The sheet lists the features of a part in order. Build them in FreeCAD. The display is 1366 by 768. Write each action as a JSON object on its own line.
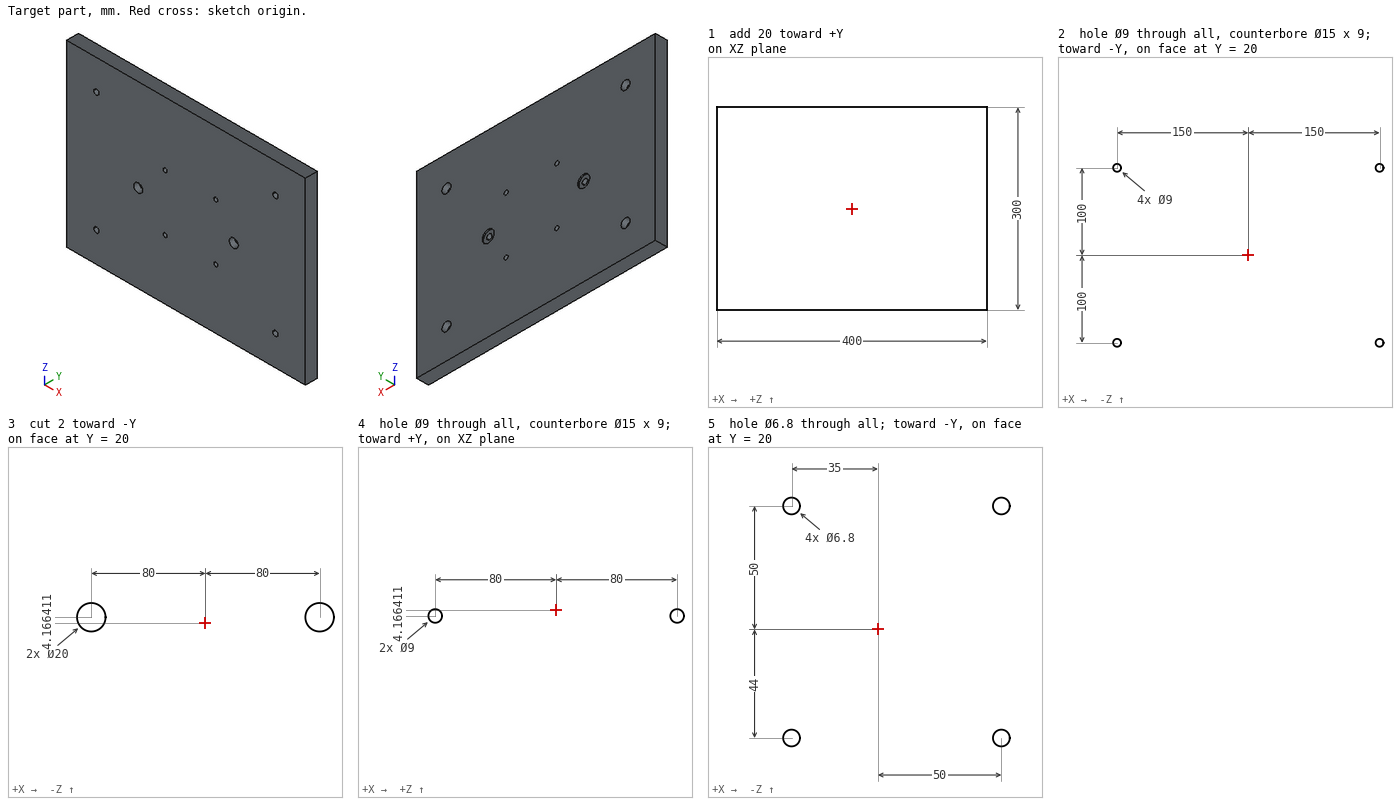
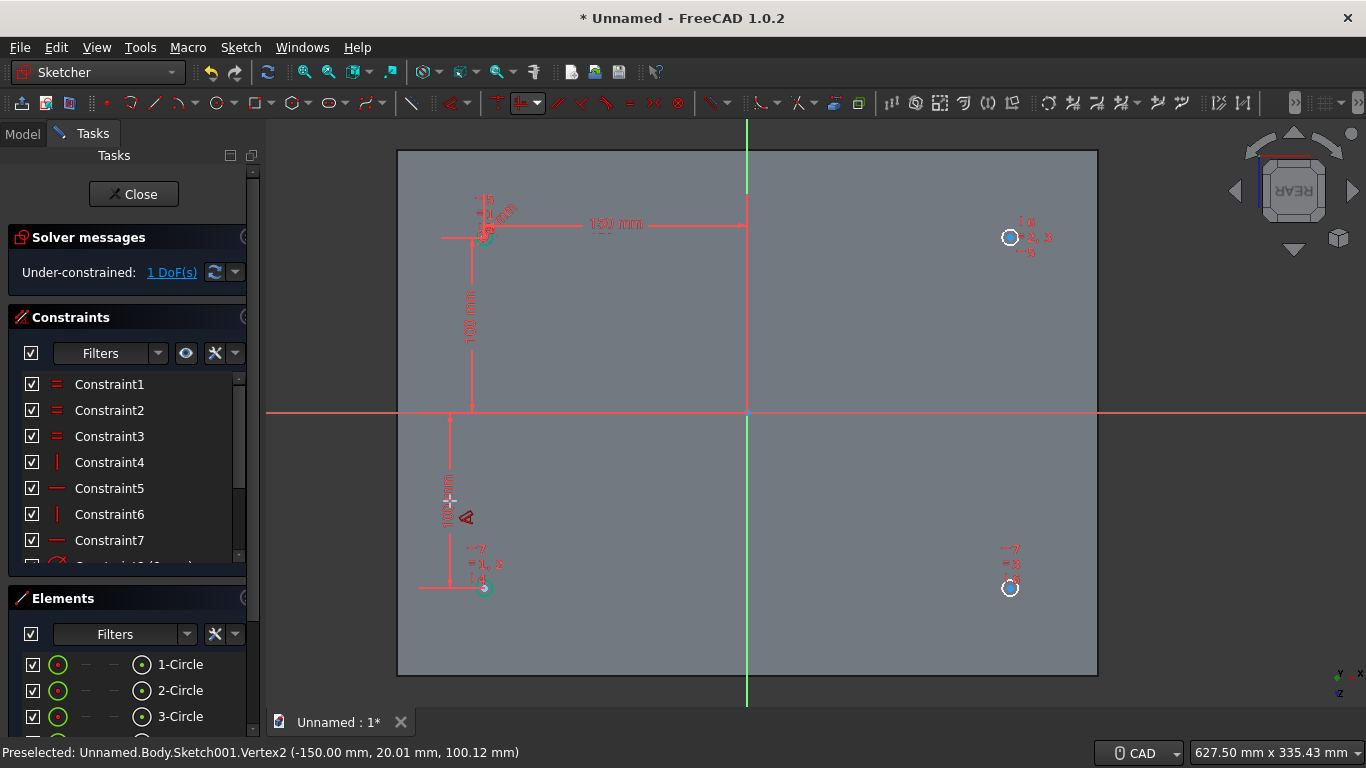
{"action": "left_click", "coordinate": [1010, 238]}
{"action": "left_click", "coordinate": [879, 204]}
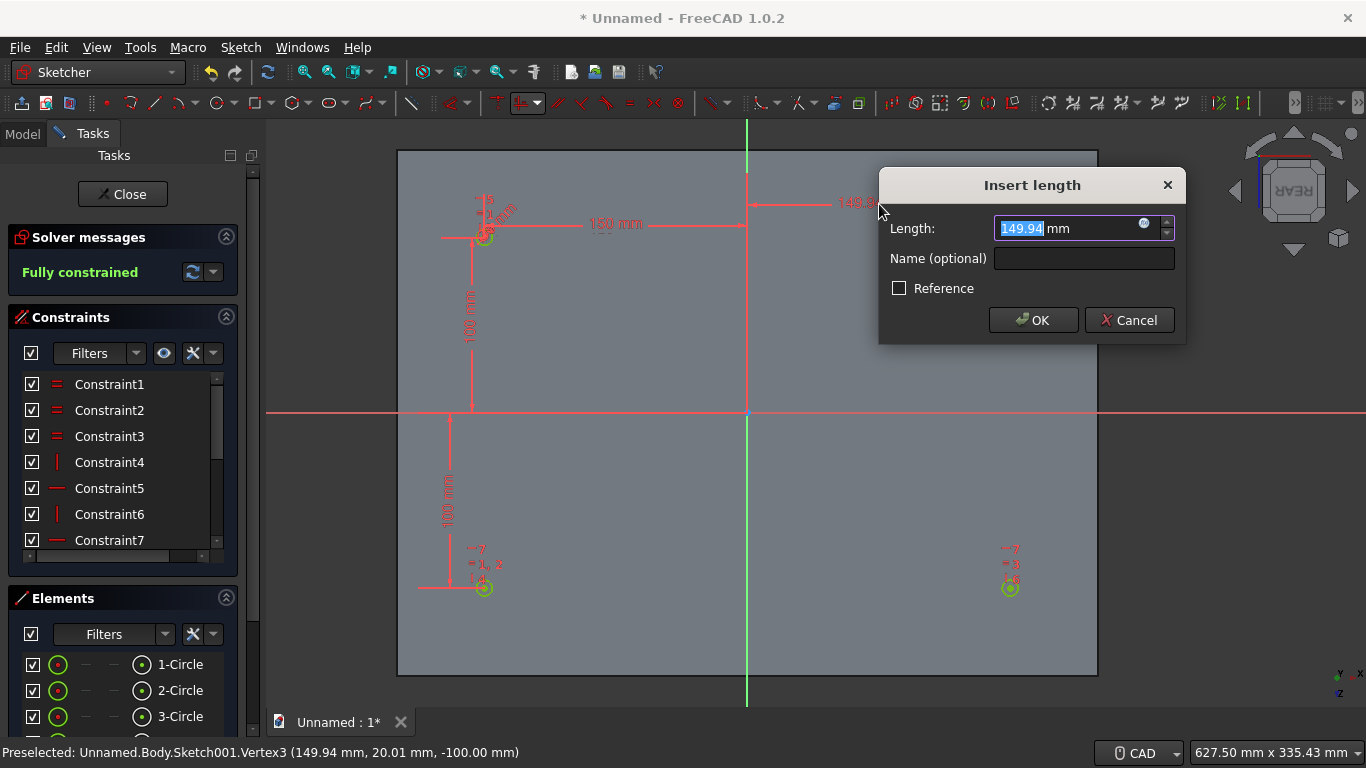
{"action": "type", "text": "150"}
{"action": "key", "text": "Return"}
{"action": "key", "text": "Escape"}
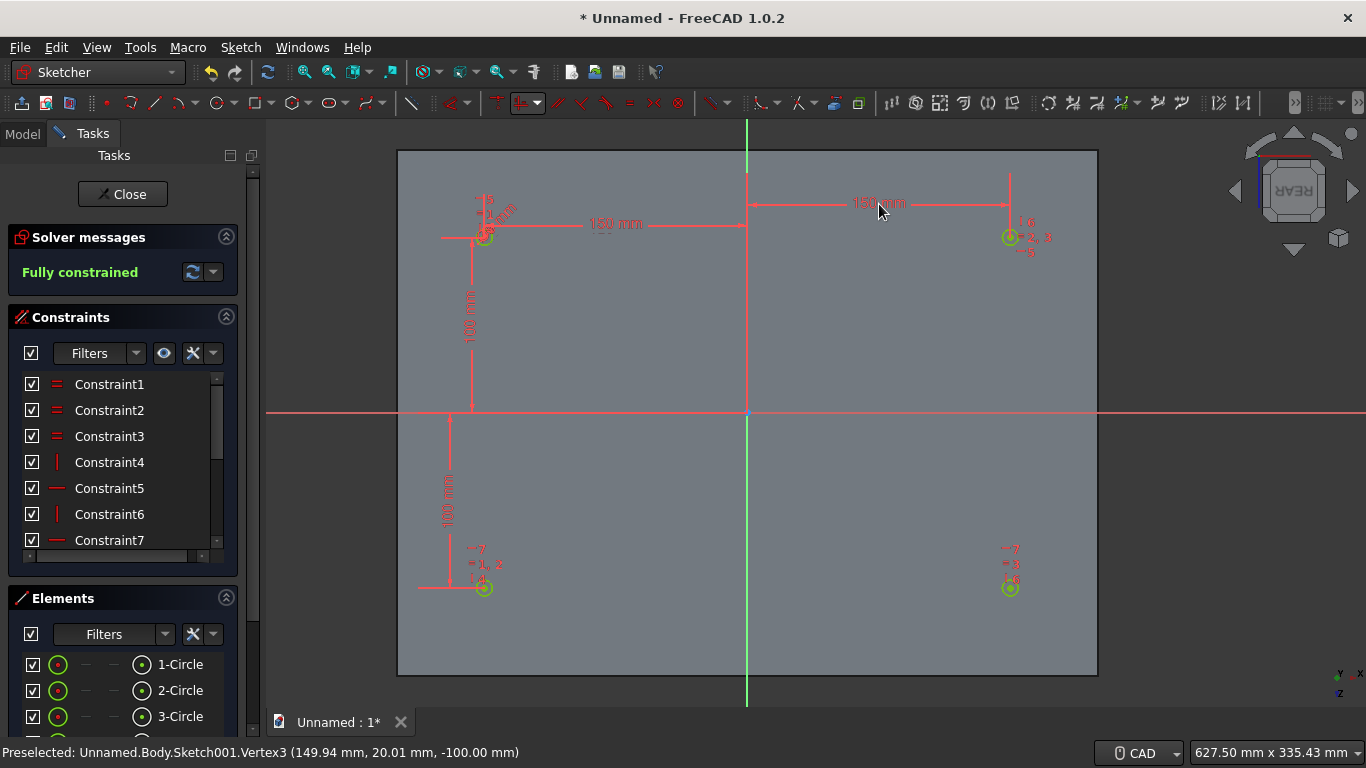
{"action": "left_click", "coordinate": [123, 194]}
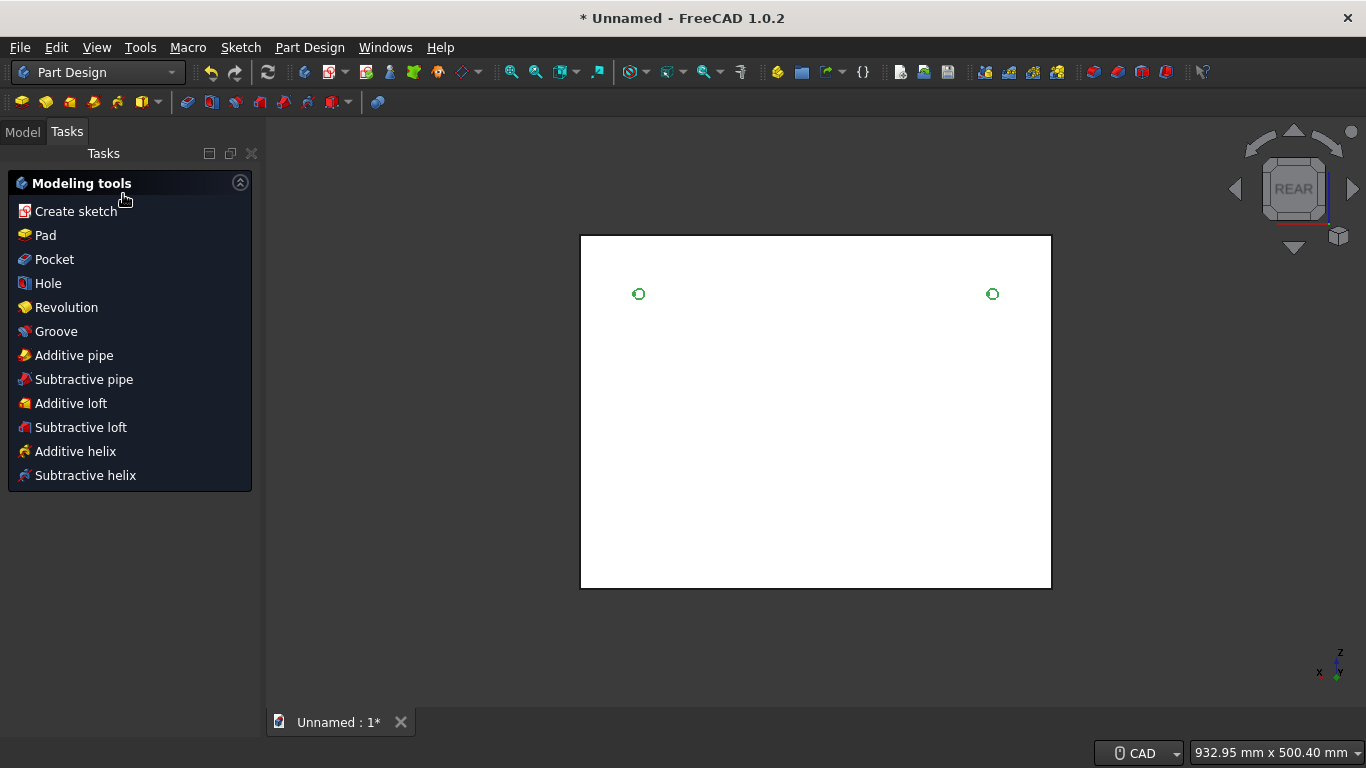
{"action": "left_click", "coordinate": [212, 102]}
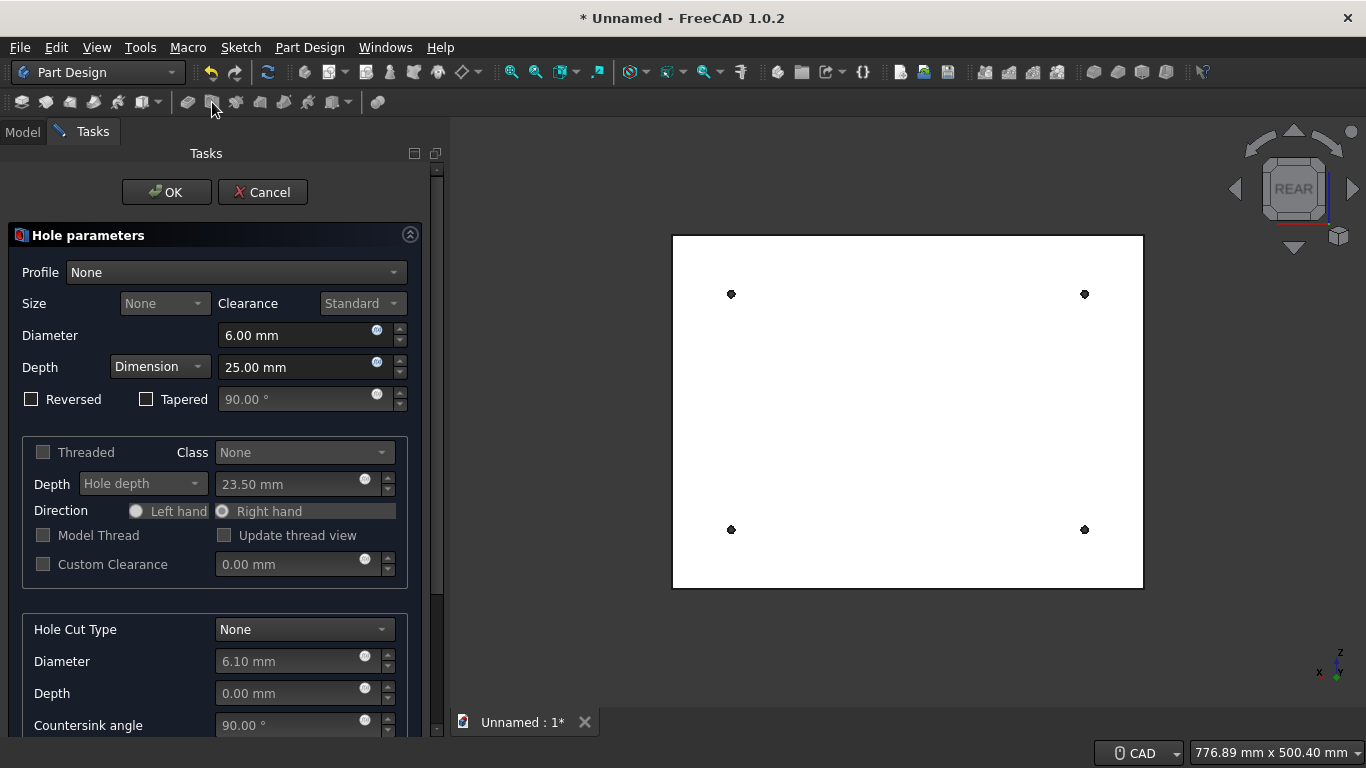
{"action": "triple_click", "coordinate": [305, 335]}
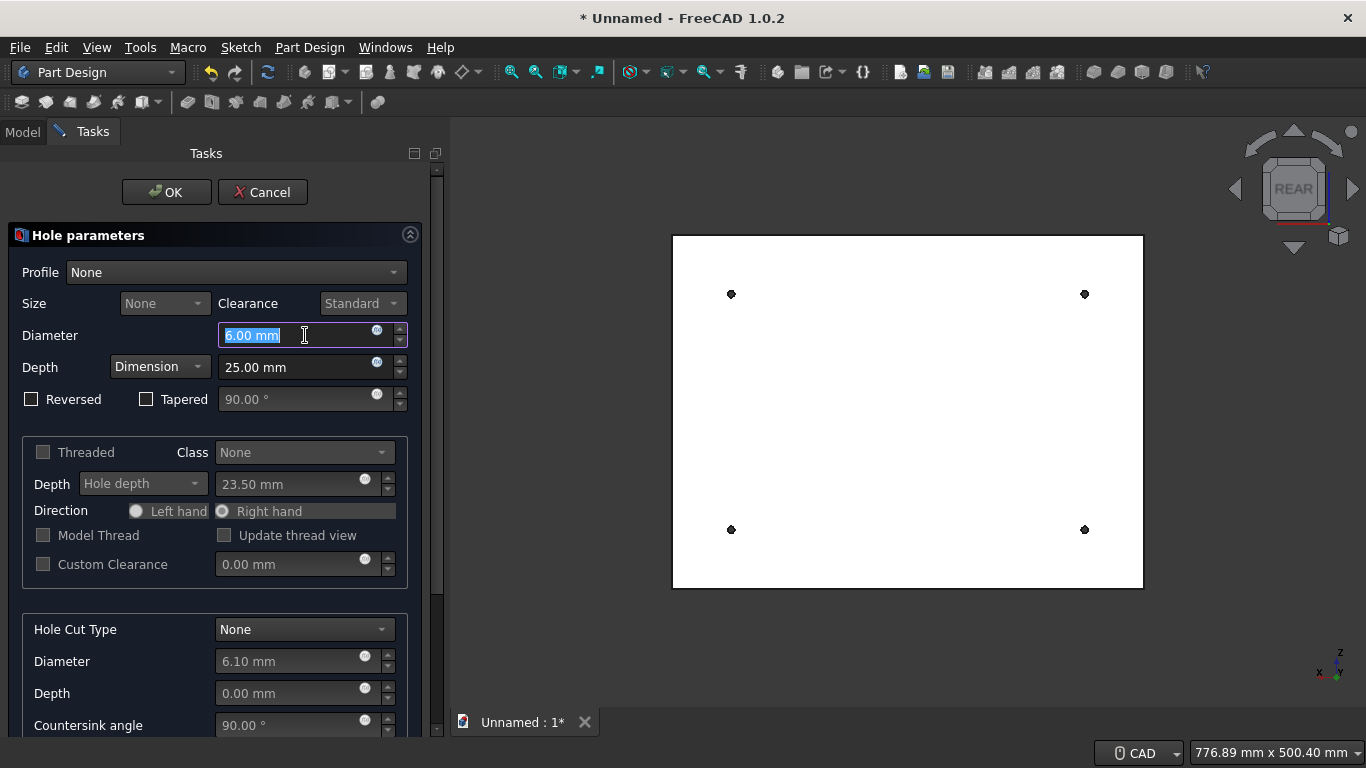
{"action": "type", "text": "9"}
{"action": "key", "text": "Tab"}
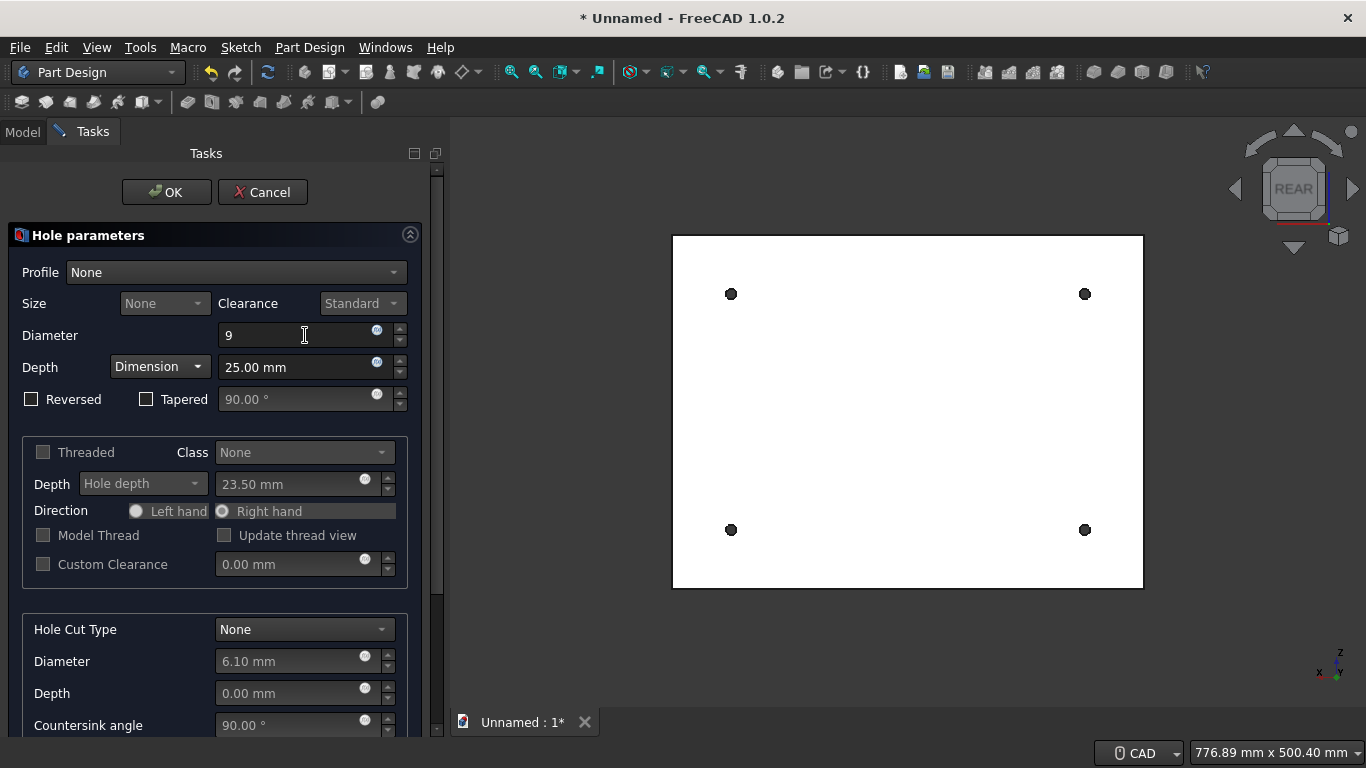
{"action": "left_click", "coordinate": [161, 366]}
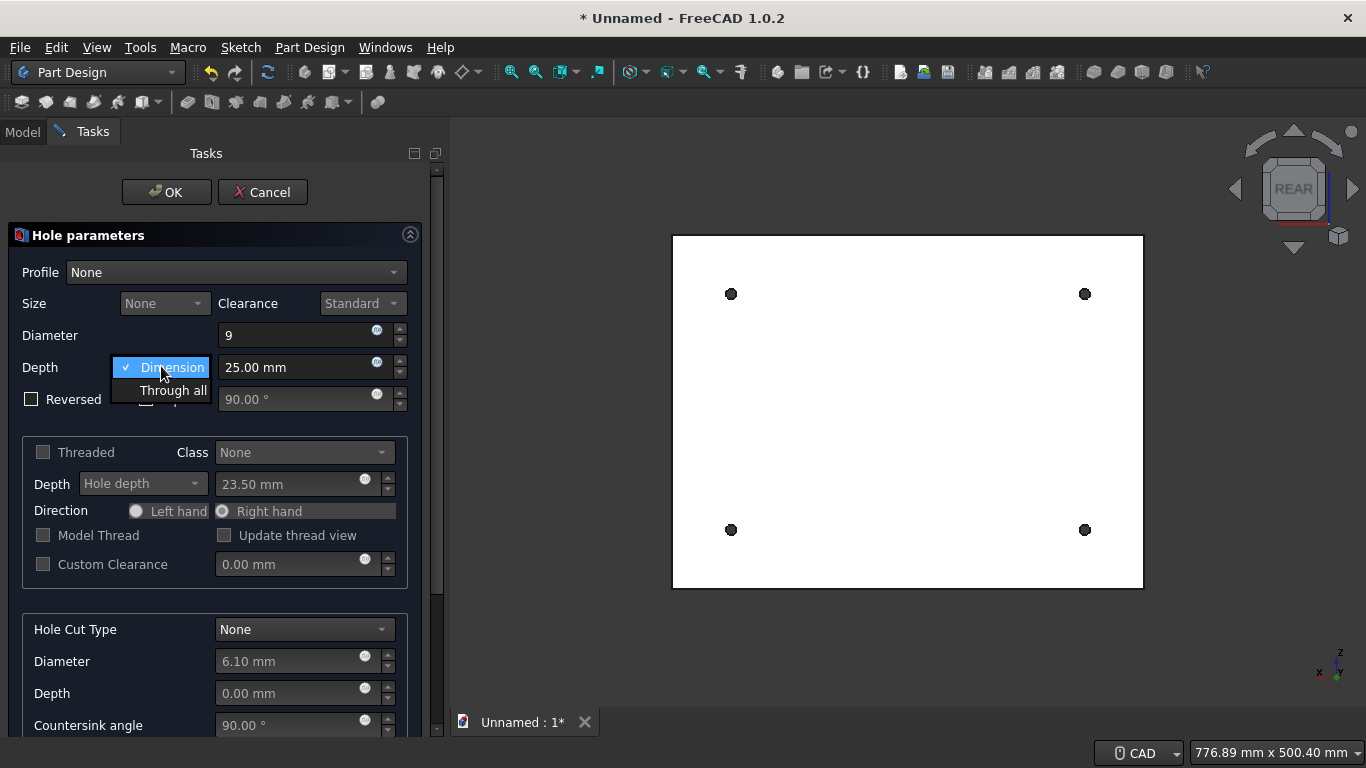
{"action": "left_click", "coordinate": [160, 390]}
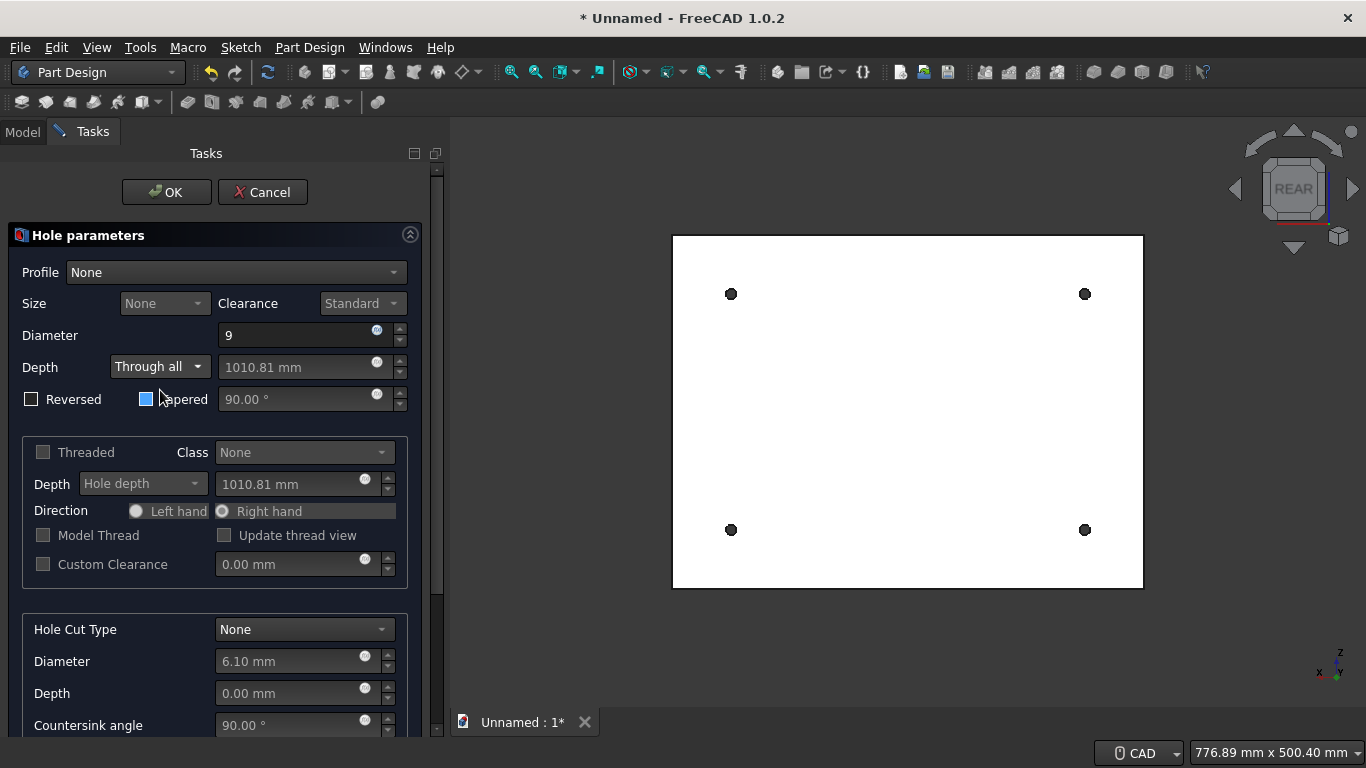
{"action": "left_click", "coordinate": [306, 630]}